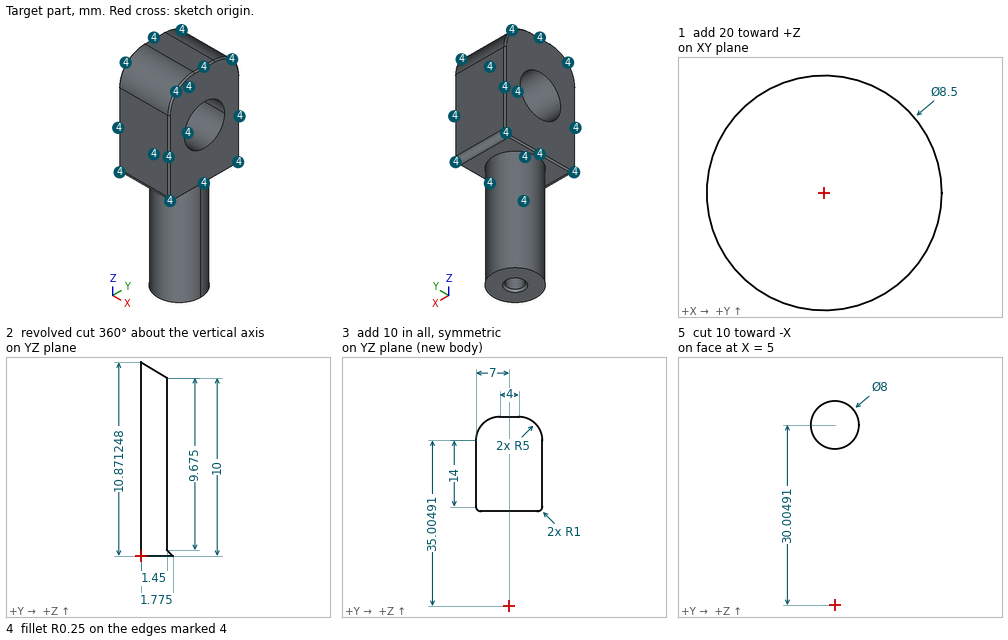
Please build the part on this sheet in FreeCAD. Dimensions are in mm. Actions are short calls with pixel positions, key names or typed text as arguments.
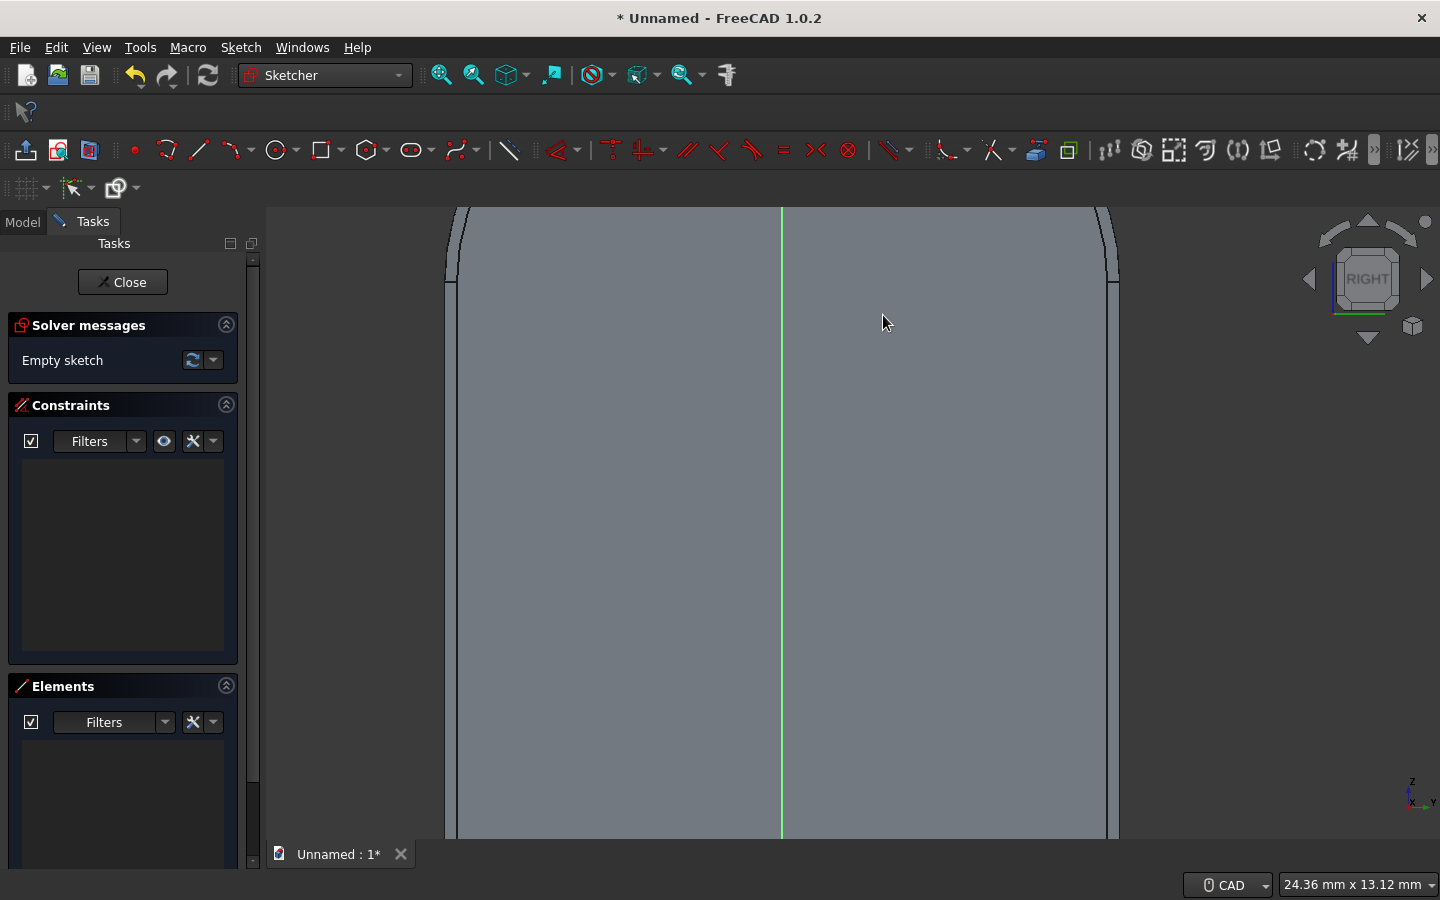
key(g)
key(c)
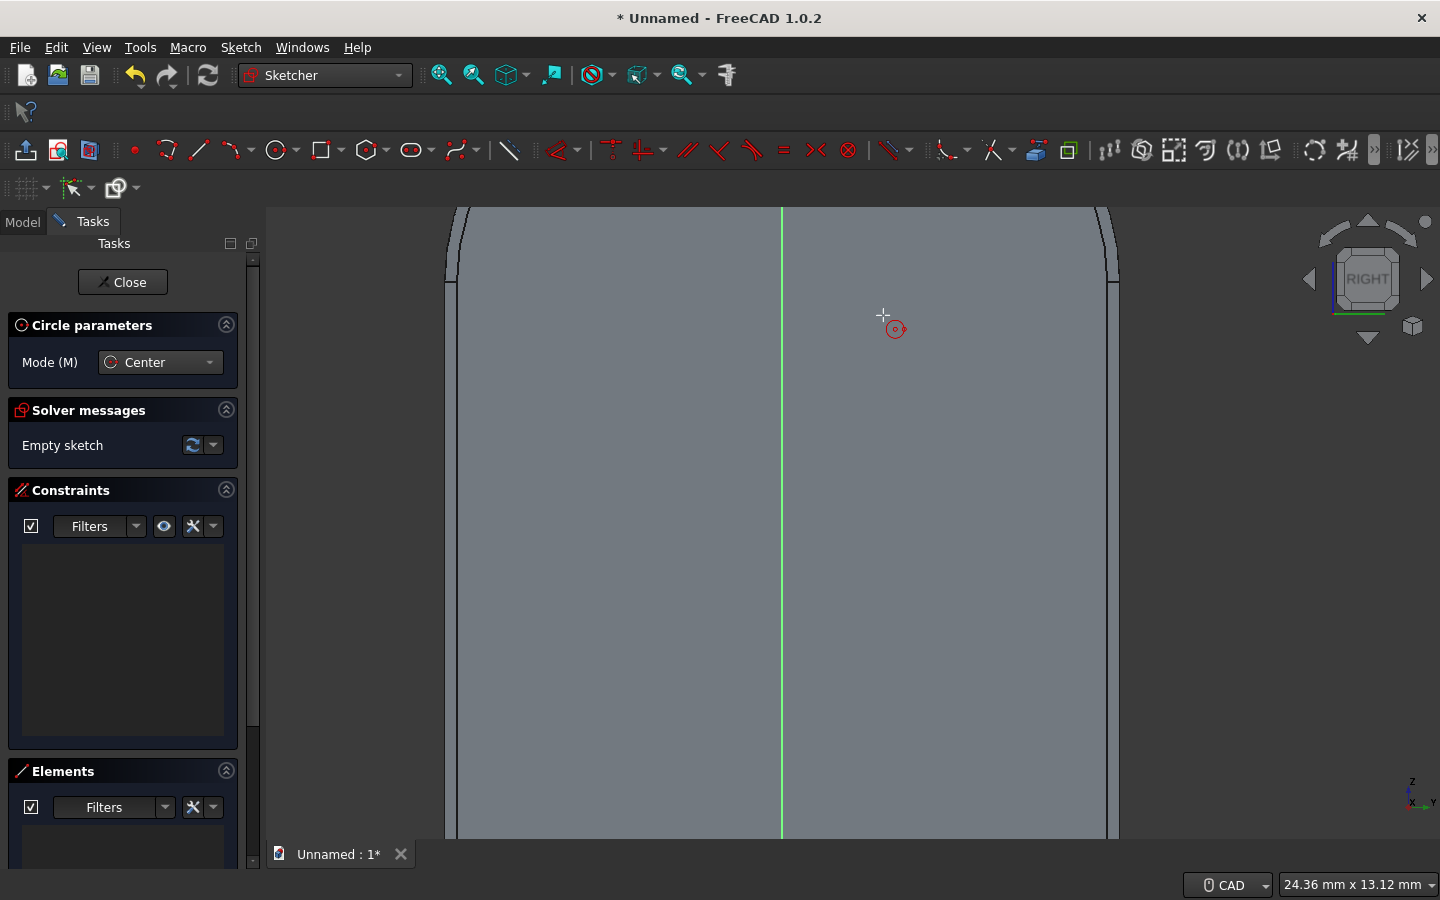
click(782, 523)
click(918, 387)
key(Escape)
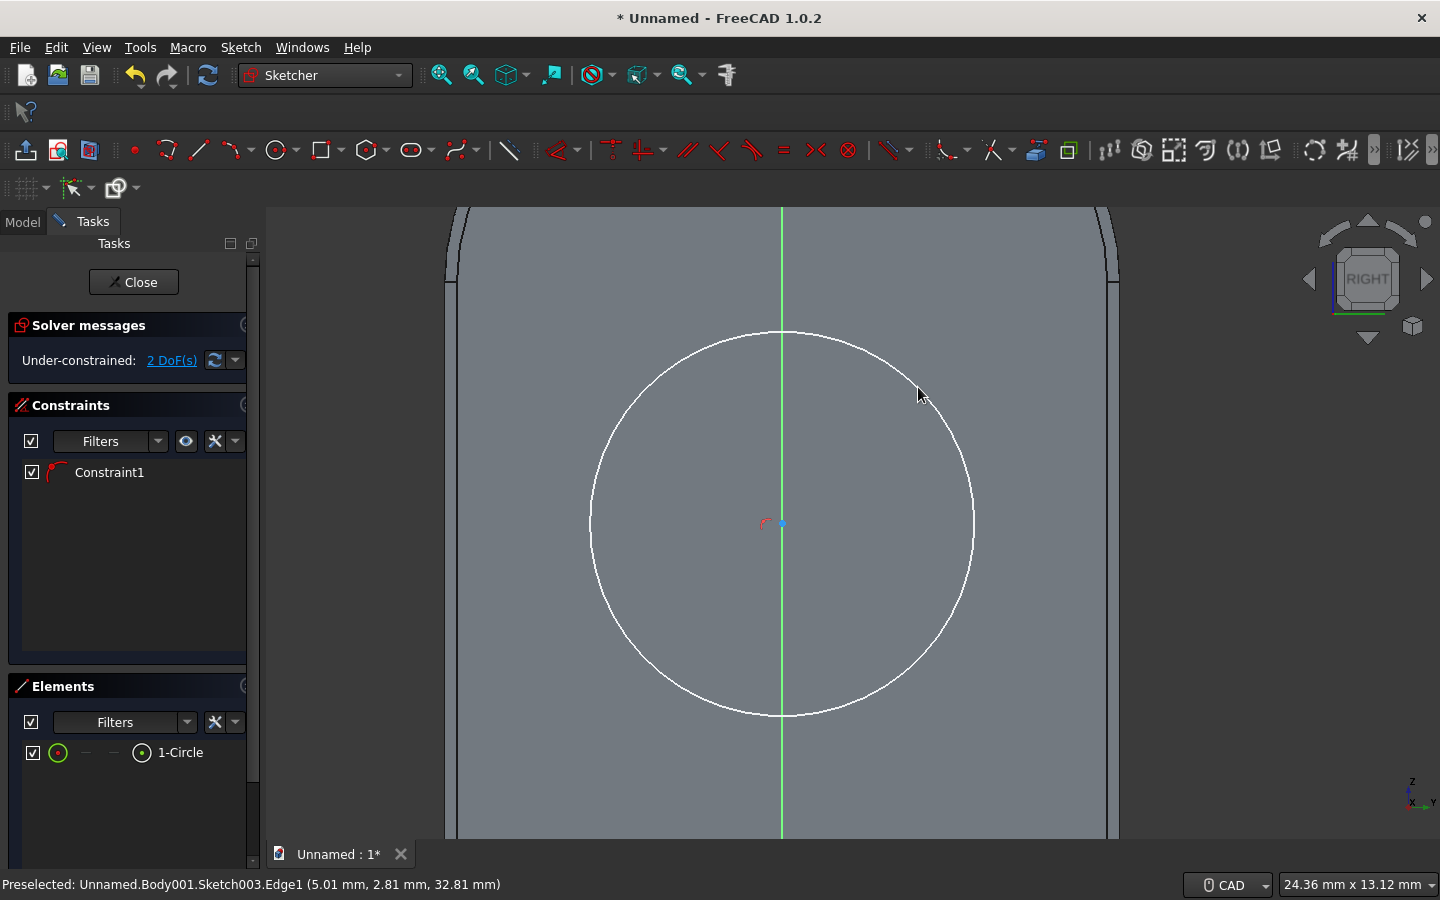
click(556, 150)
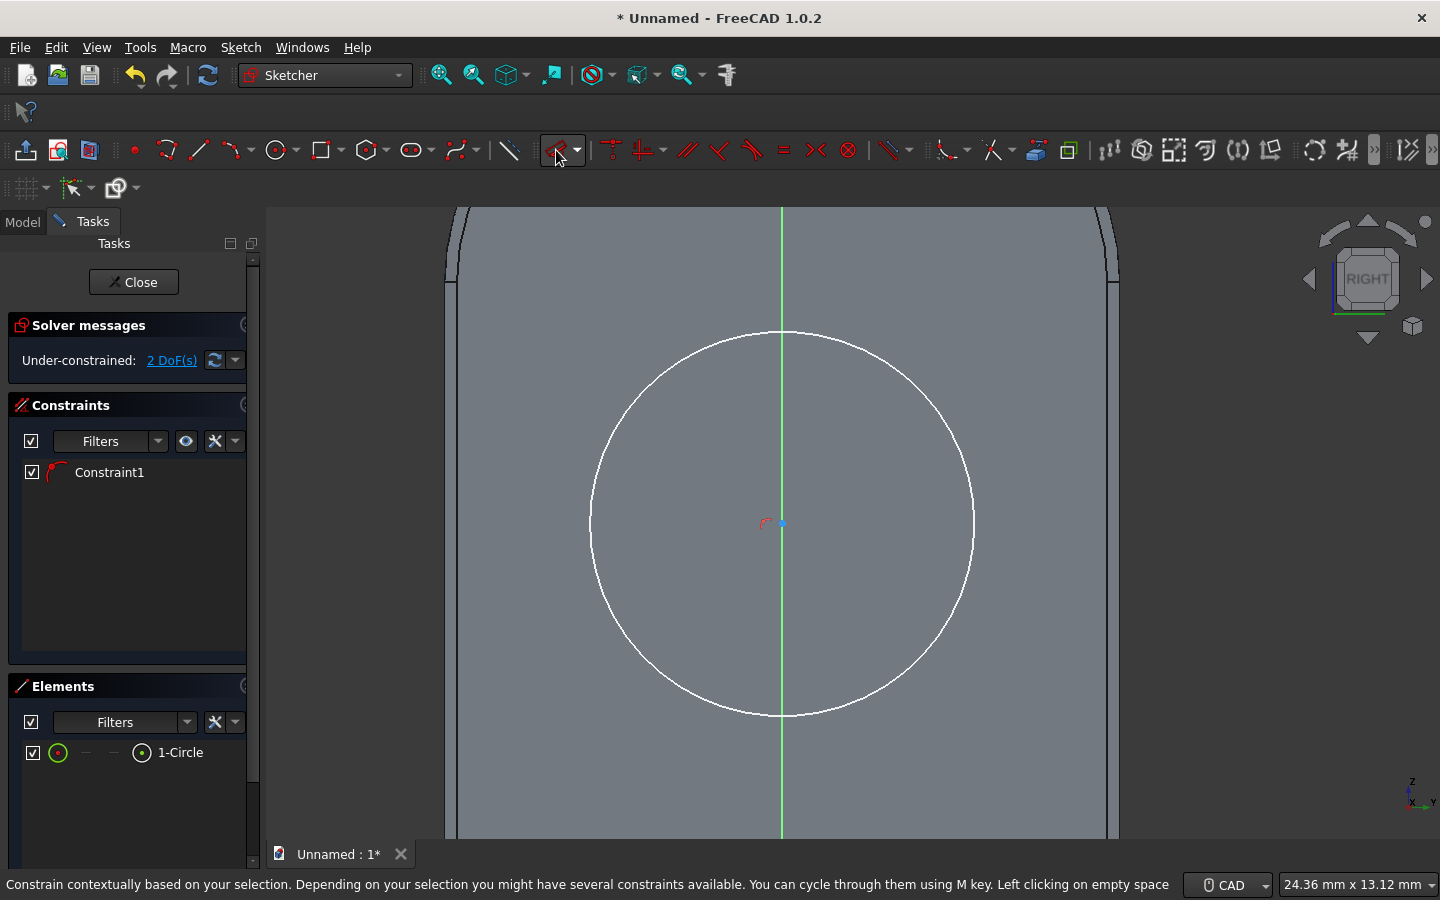
click(918, 388)
click(941, 365)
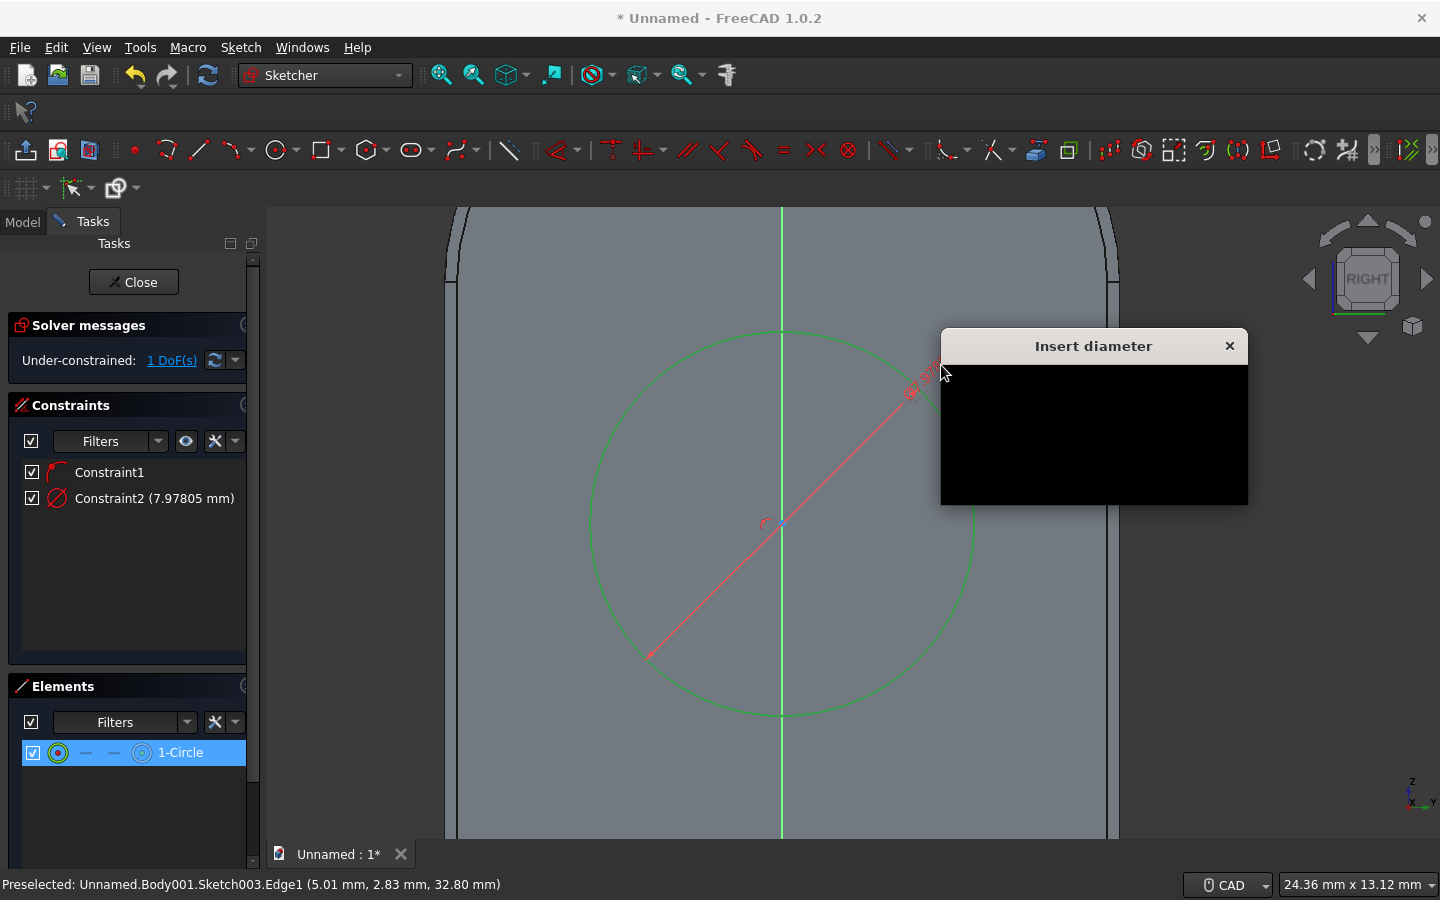
text(8)
key(Return)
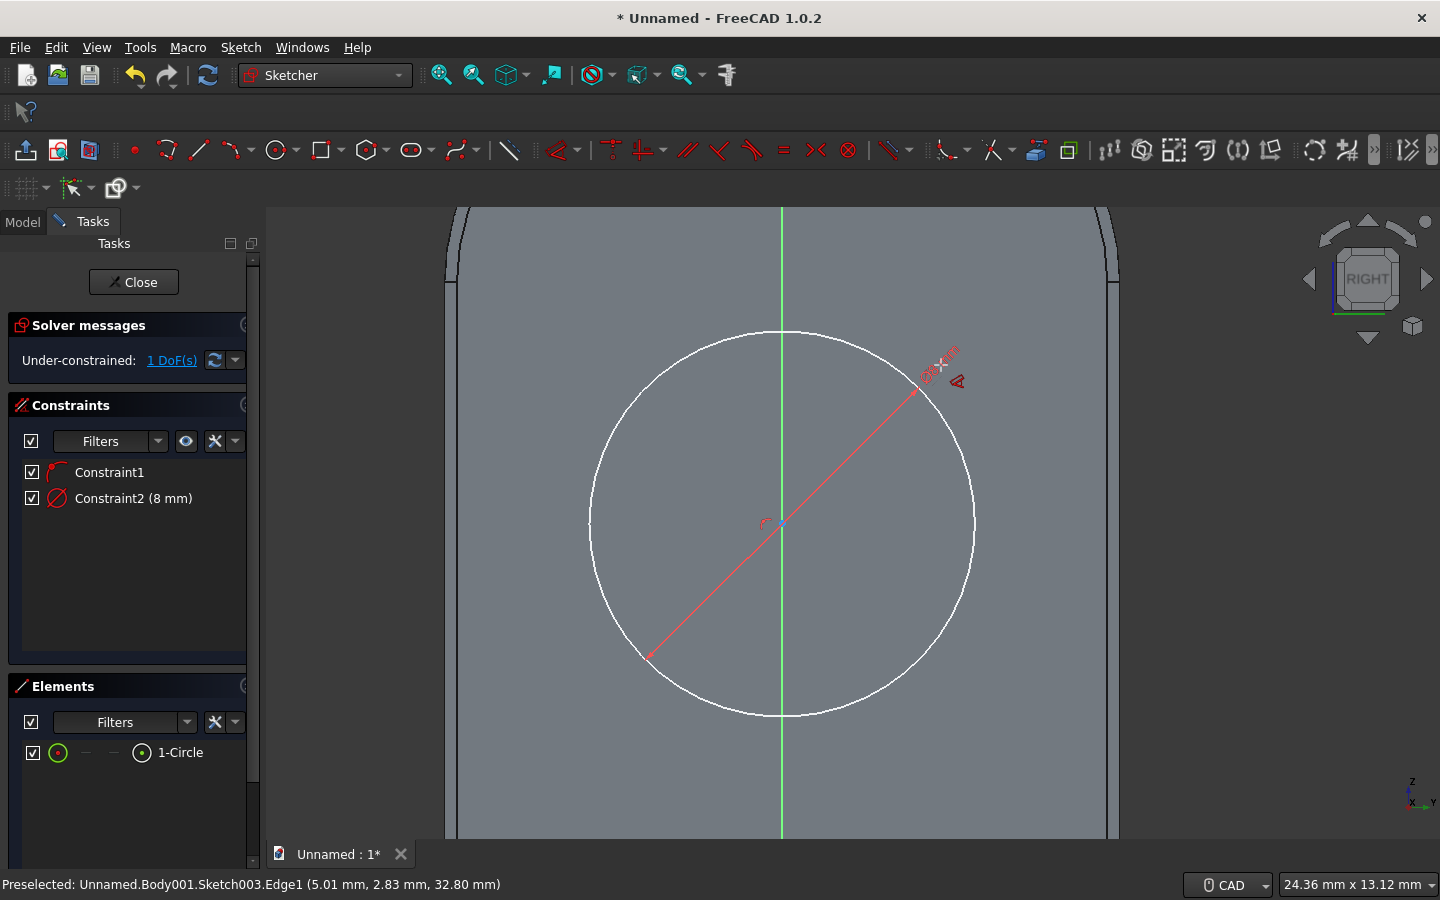
click(782, 524)
click(816, 667)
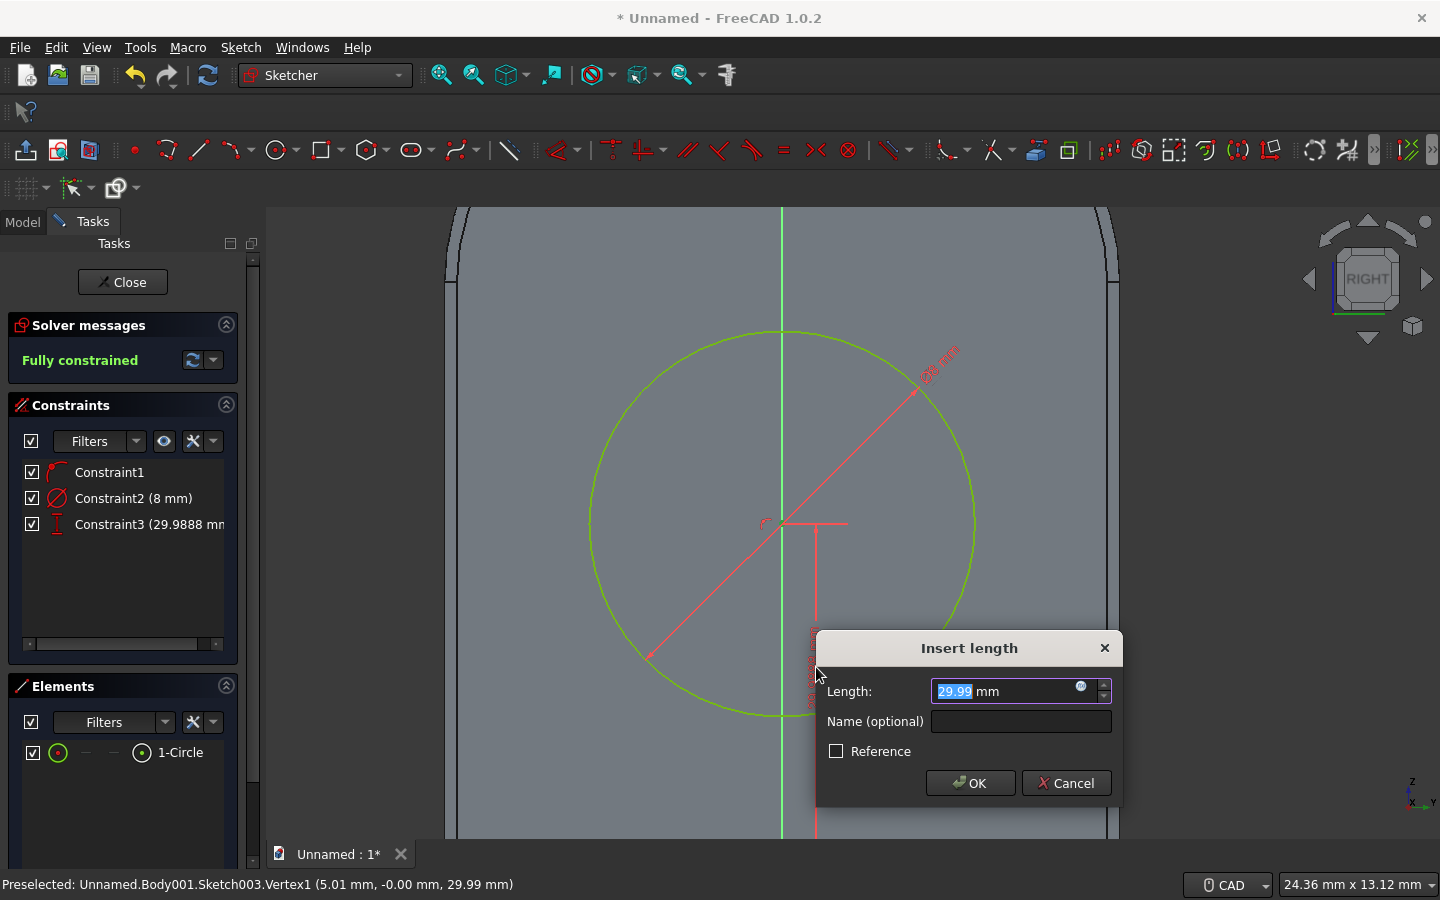
text(30.00491)
key(Return)
key(Escape)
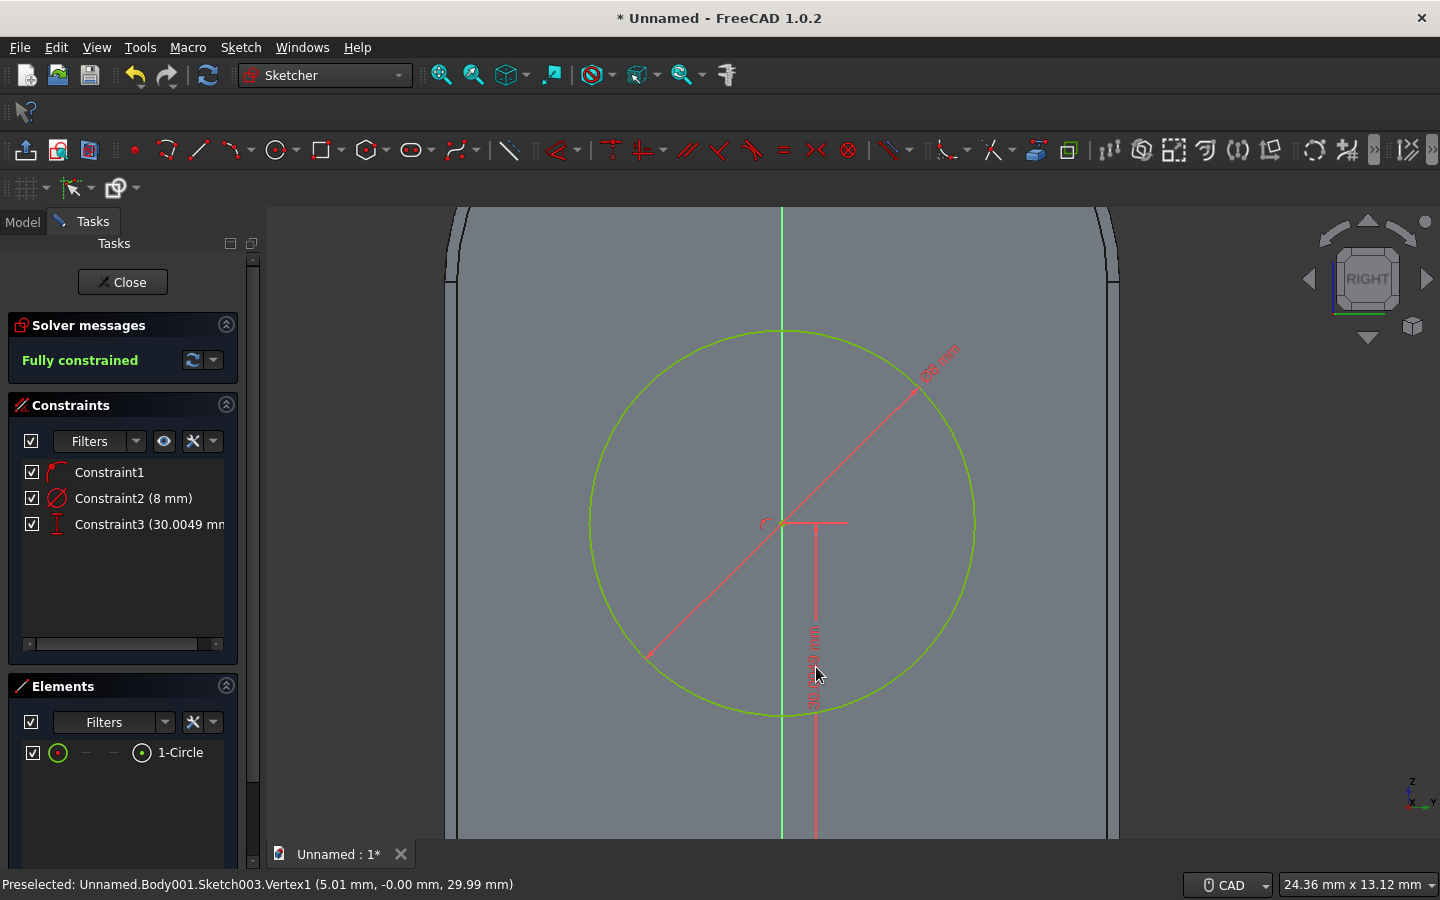
click(123, 282)